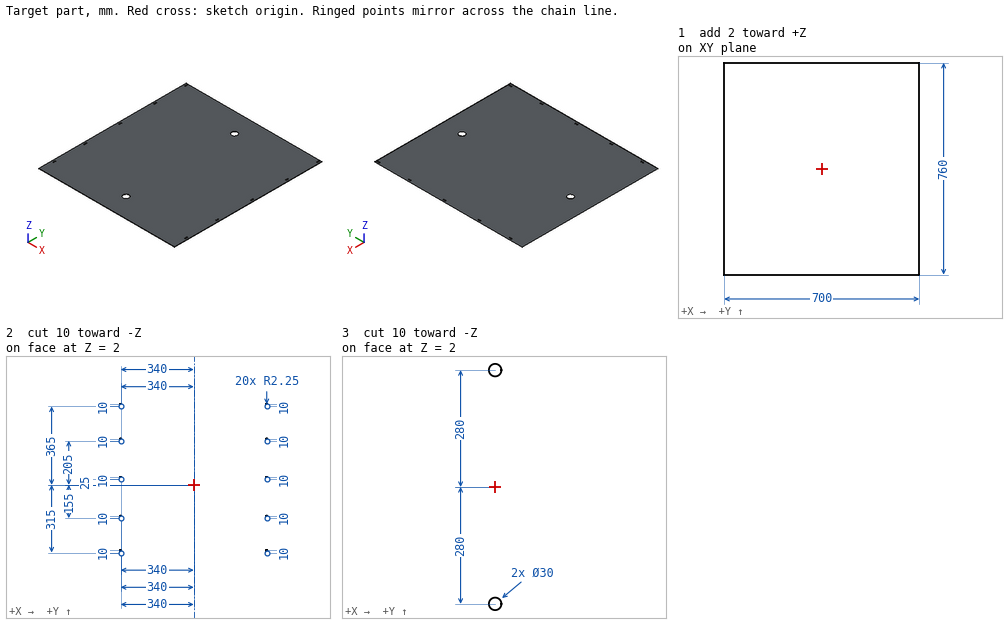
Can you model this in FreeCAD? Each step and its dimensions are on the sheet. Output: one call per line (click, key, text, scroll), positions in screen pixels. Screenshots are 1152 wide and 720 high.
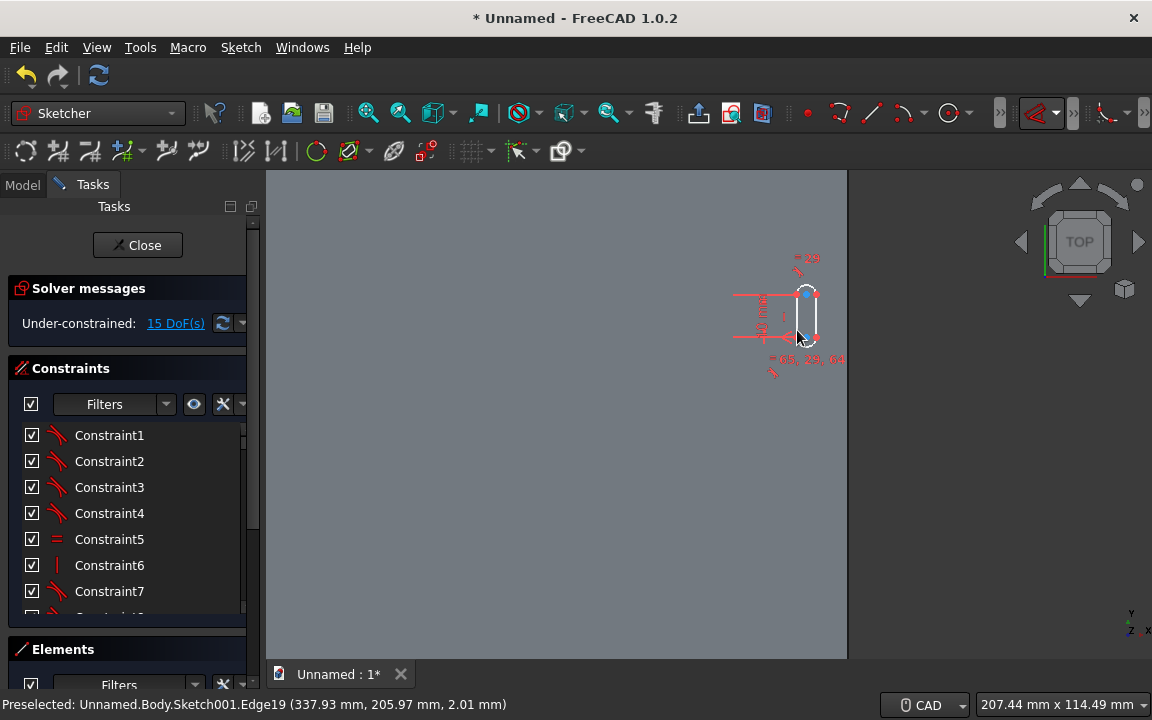
scroll(801, 331, down, 11)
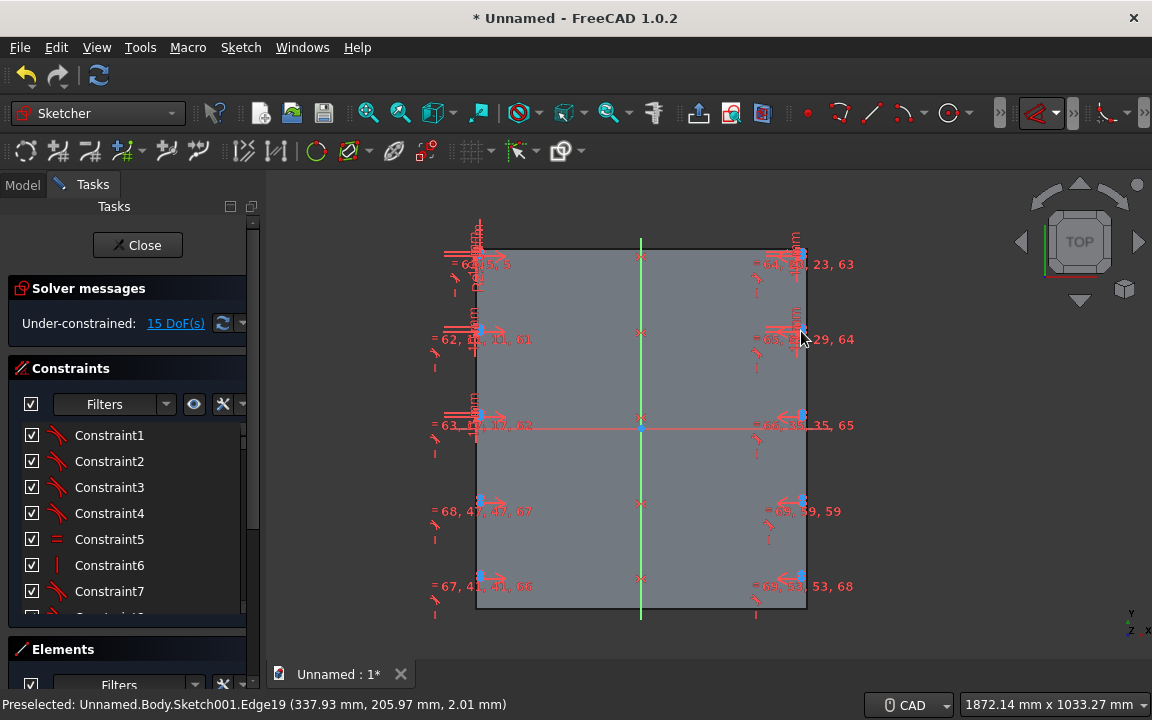
scroll(801, 416, up, 12)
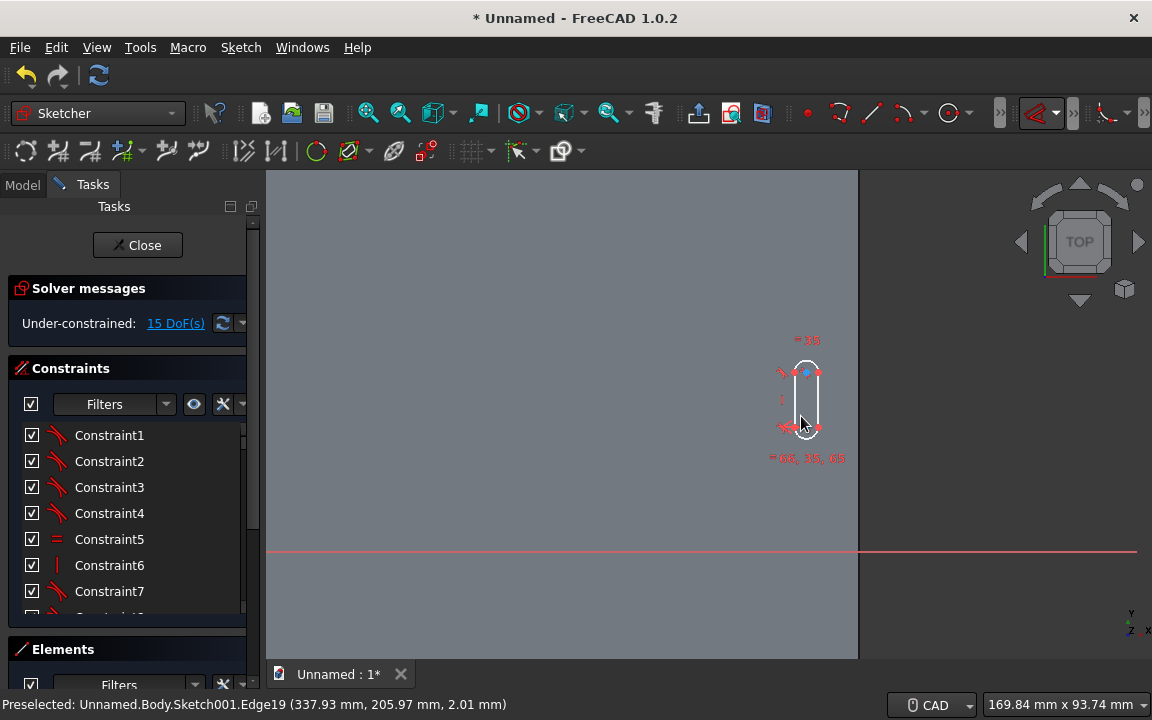
click(795, 411)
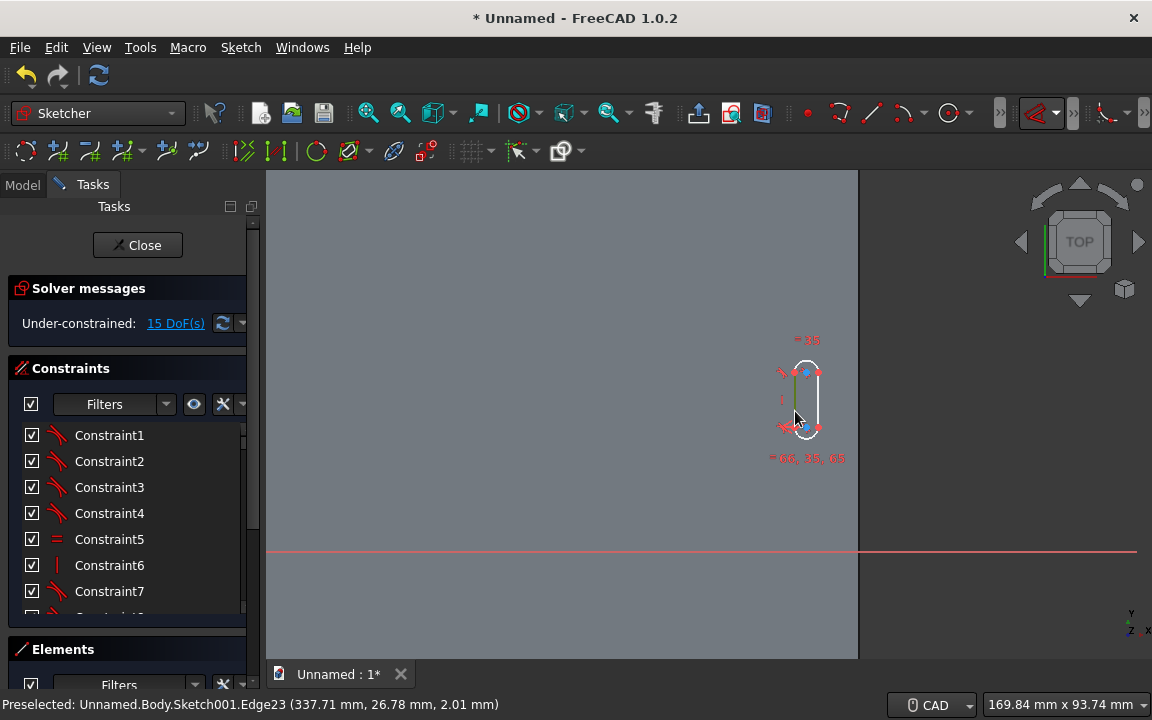
click(1058, 114)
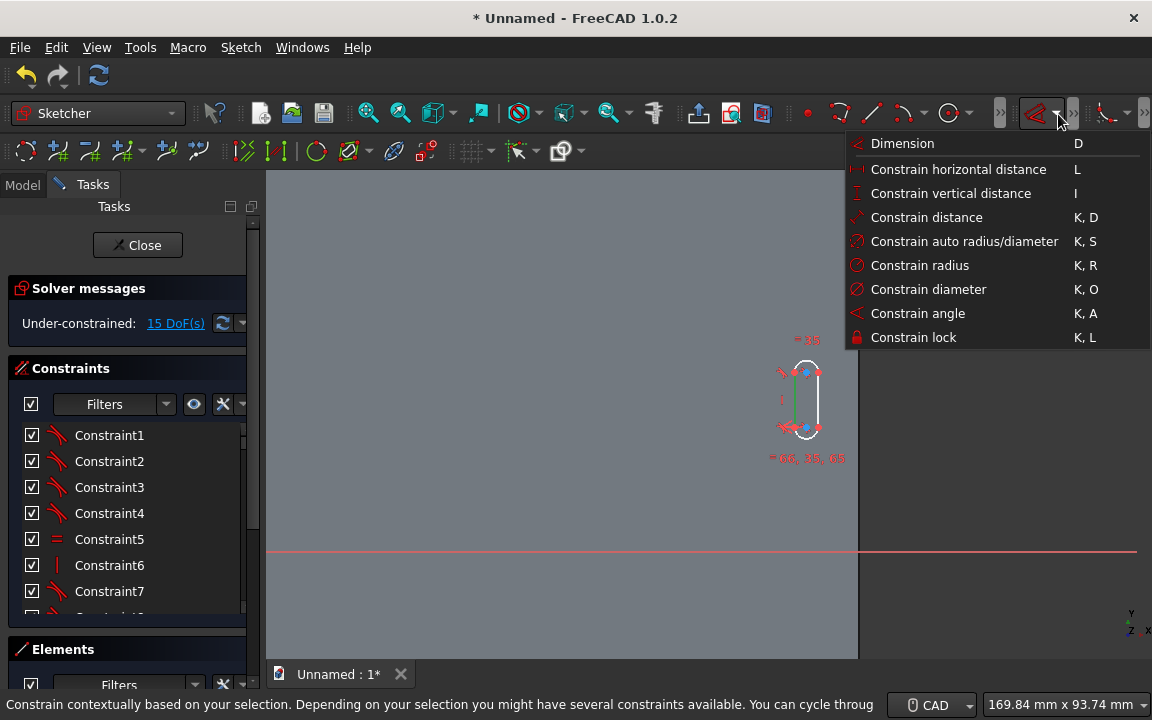
click(998, 193)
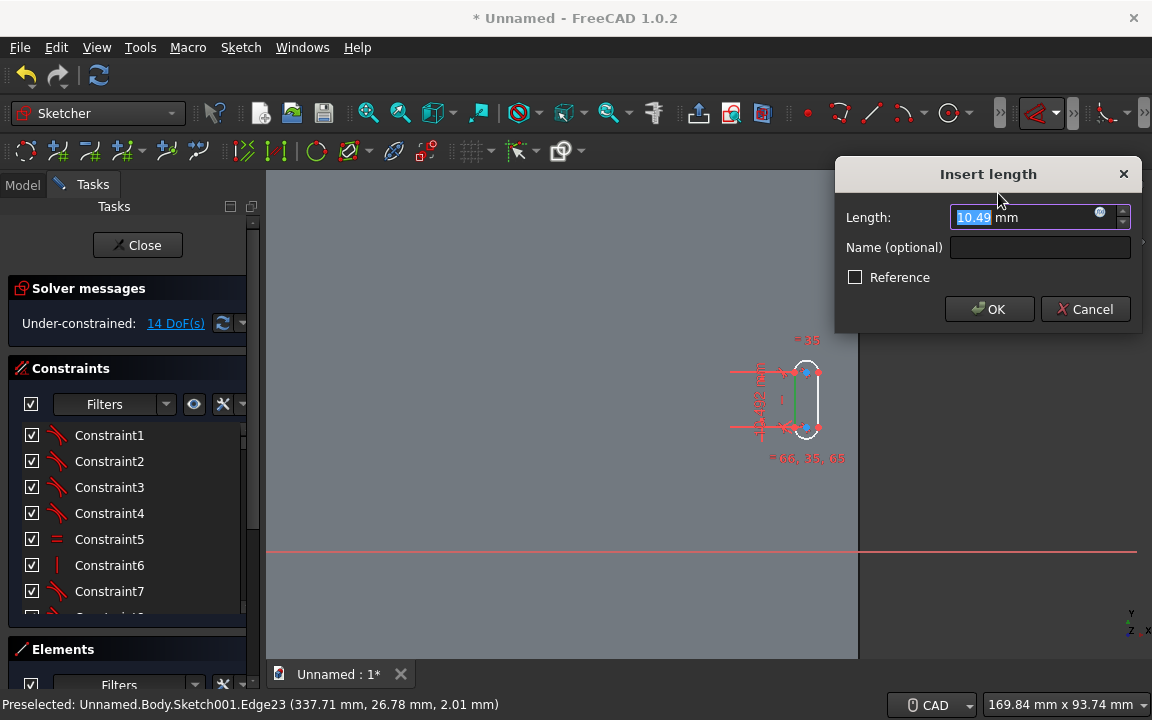
text(10)
key(Return)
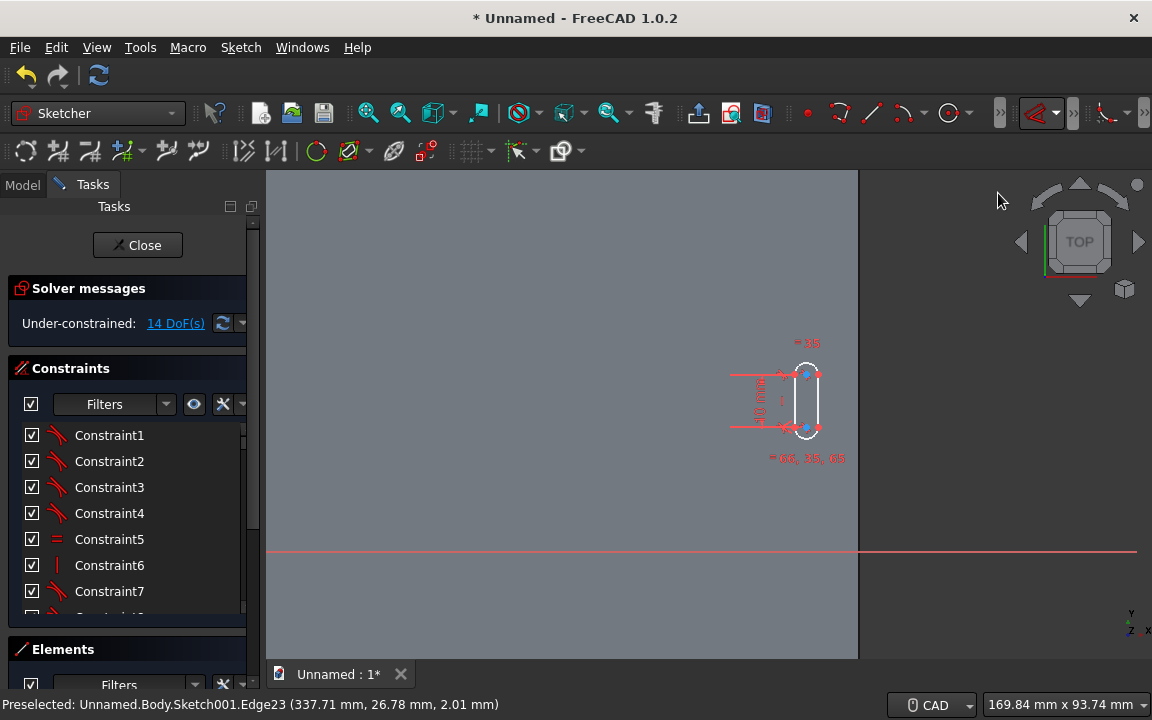
scroll(801, 416, down, 12)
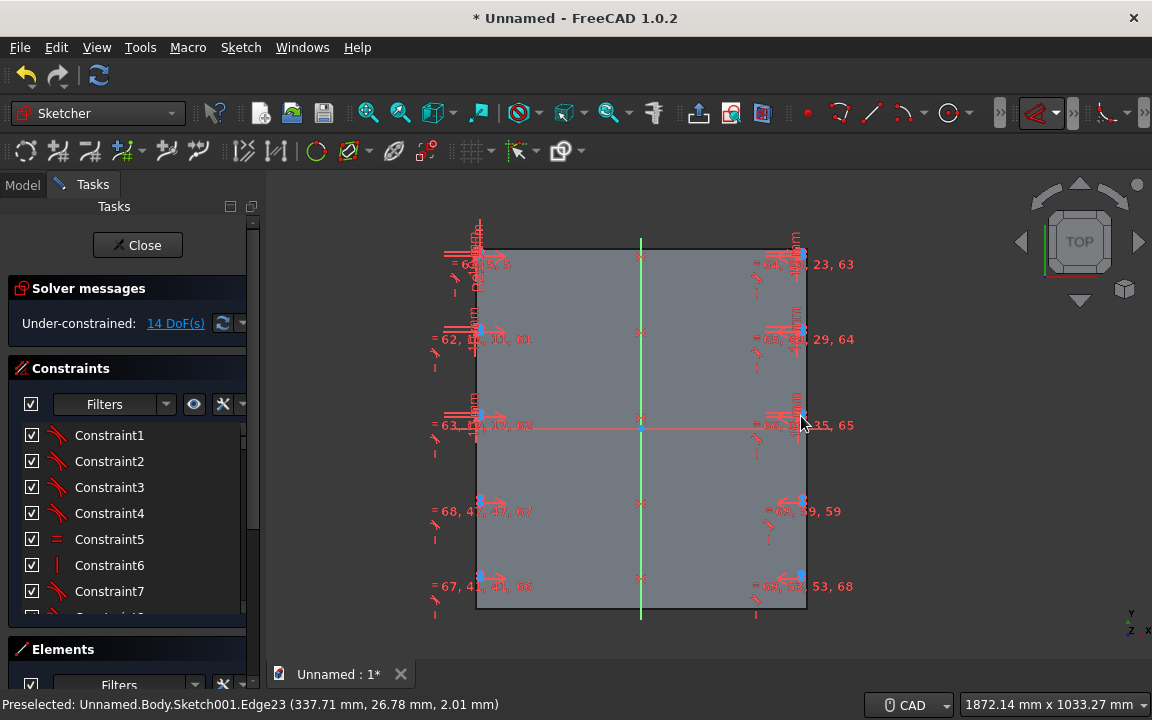
scroll(480, 577, up, 11)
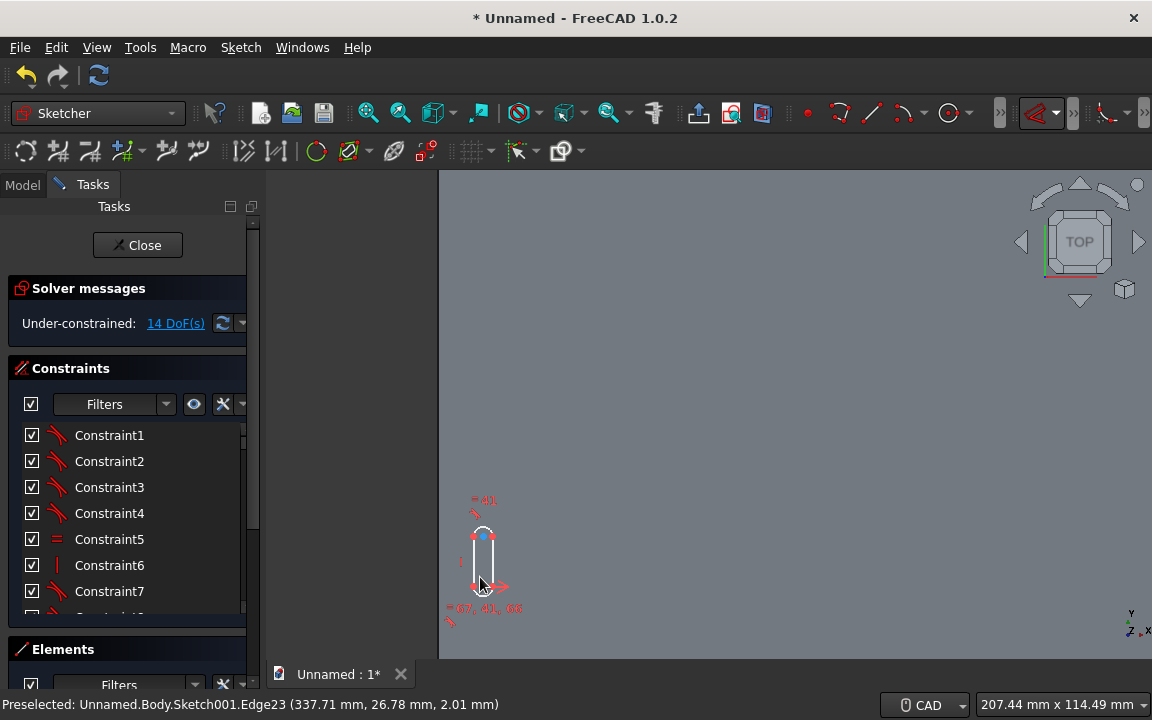
click(474, 572)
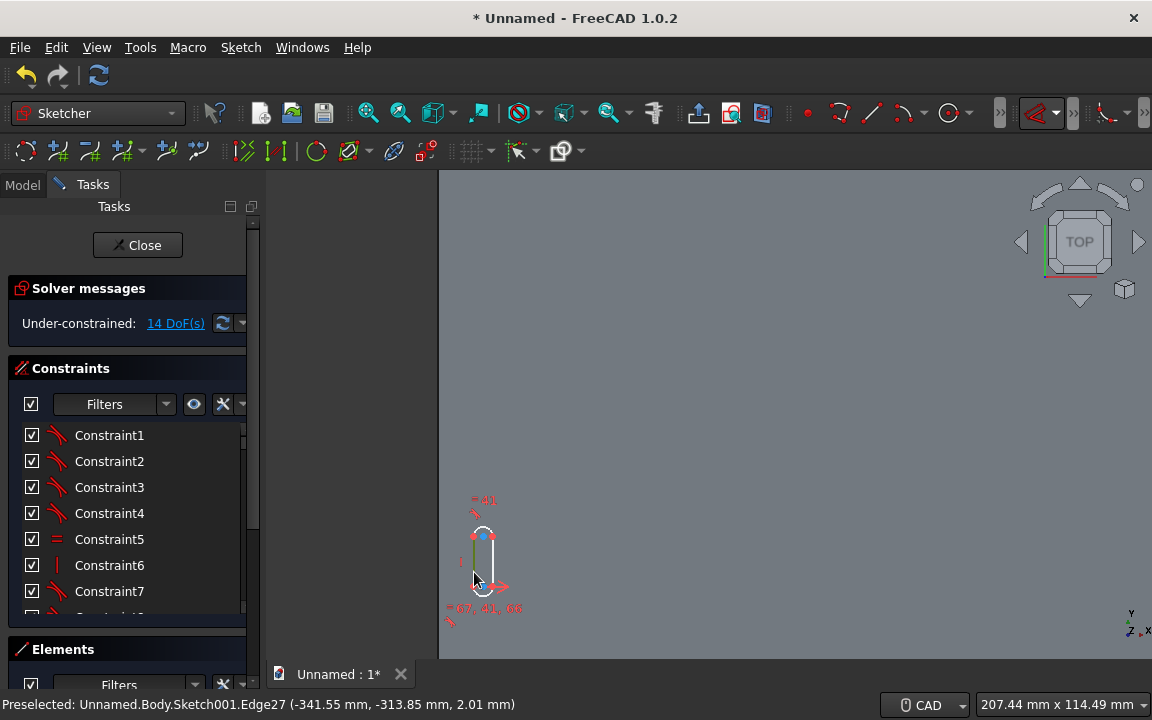
key(i)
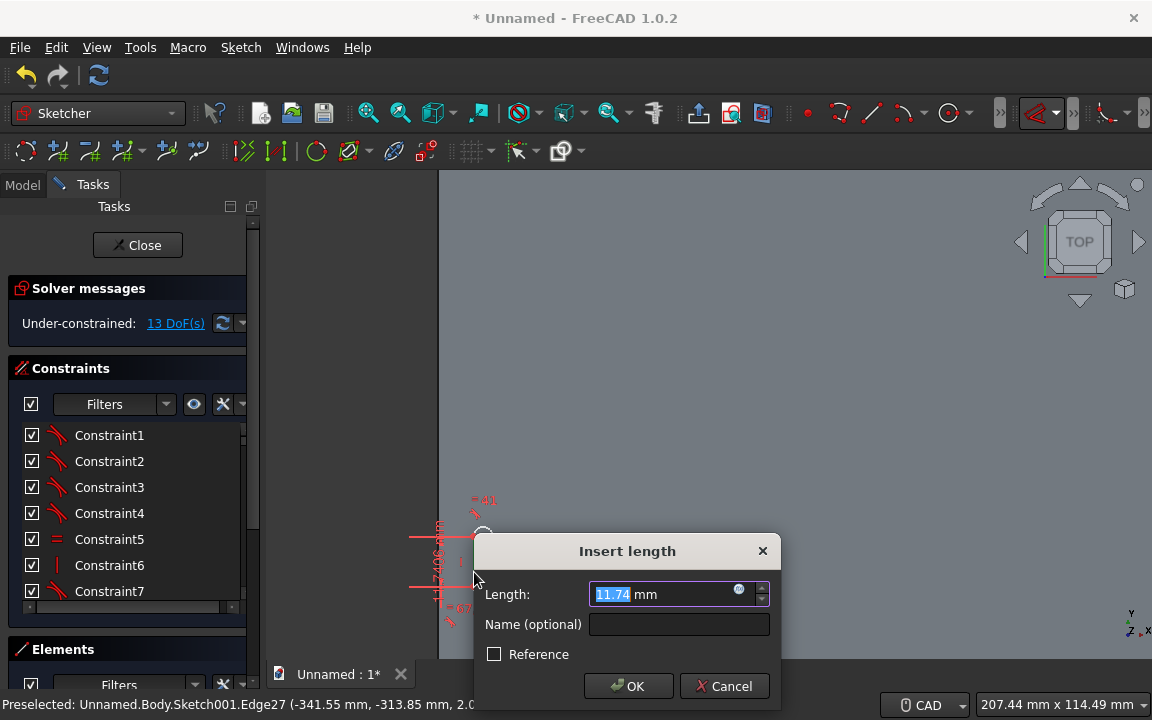
text(10)
key(Return)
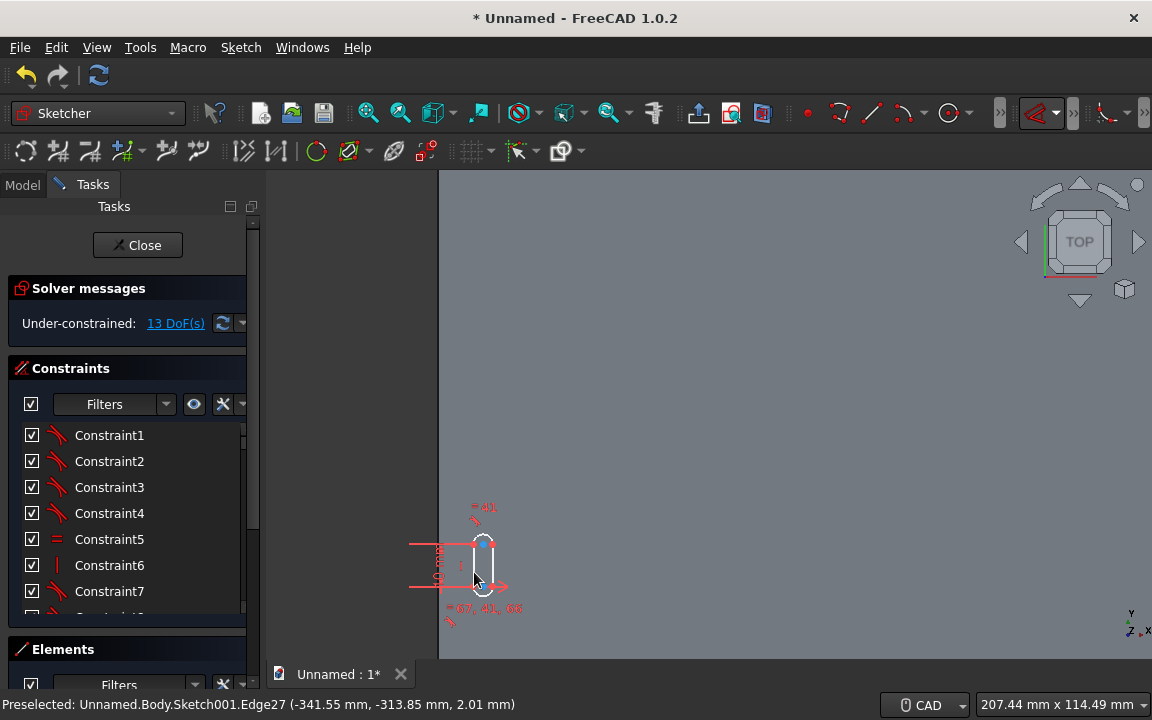
scroll(480, 578, down, 11)